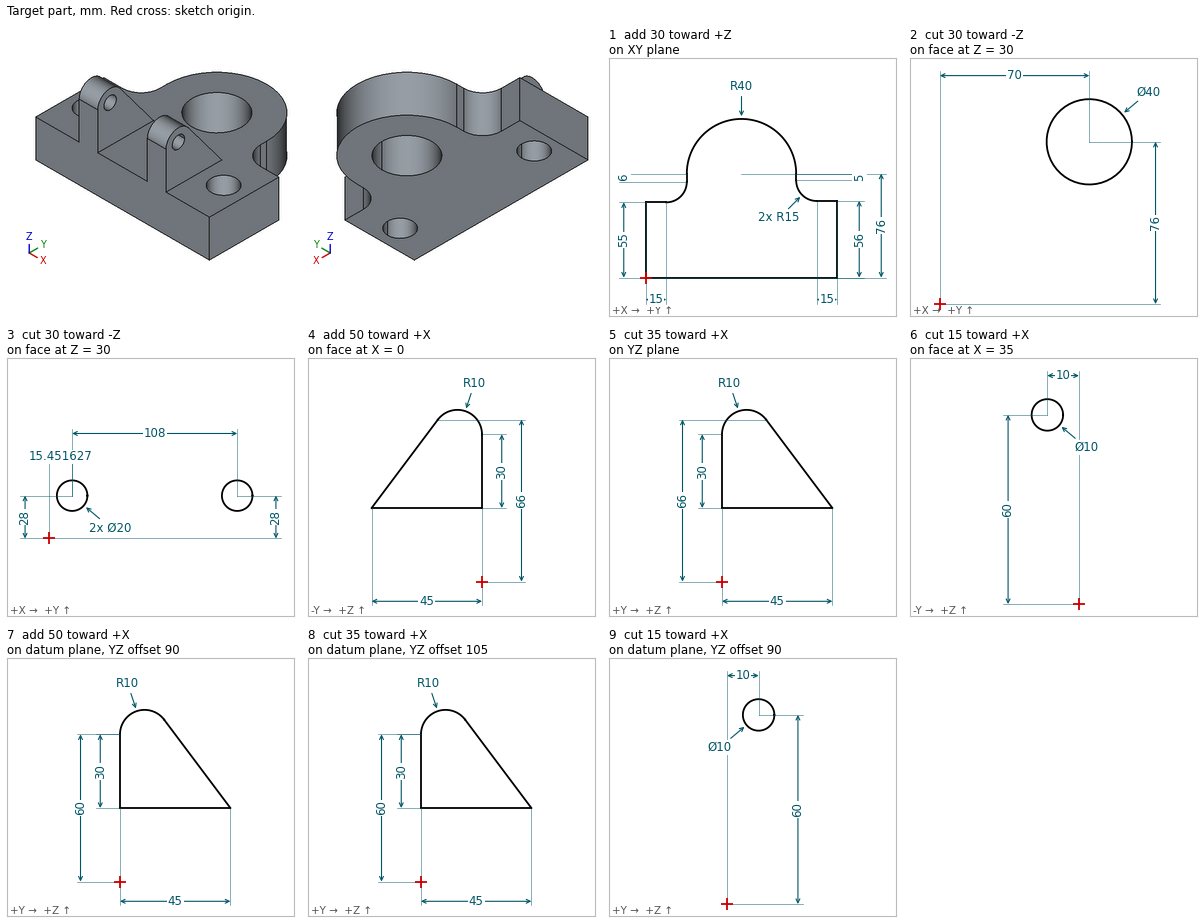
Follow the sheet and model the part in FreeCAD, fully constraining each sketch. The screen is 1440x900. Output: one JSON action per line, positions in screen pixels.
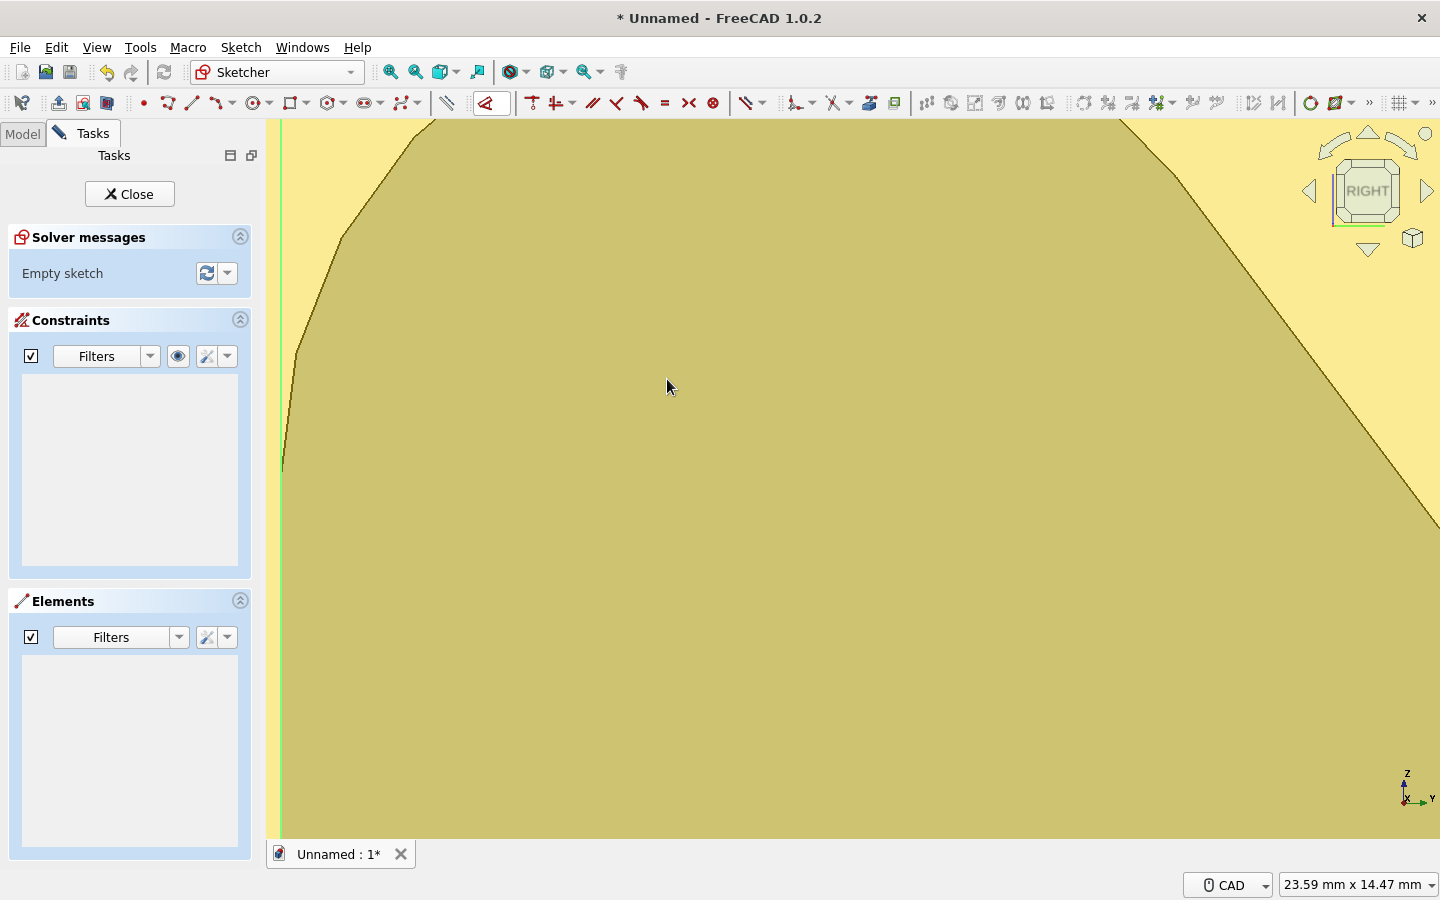
{"action": "key", "text": "g c"}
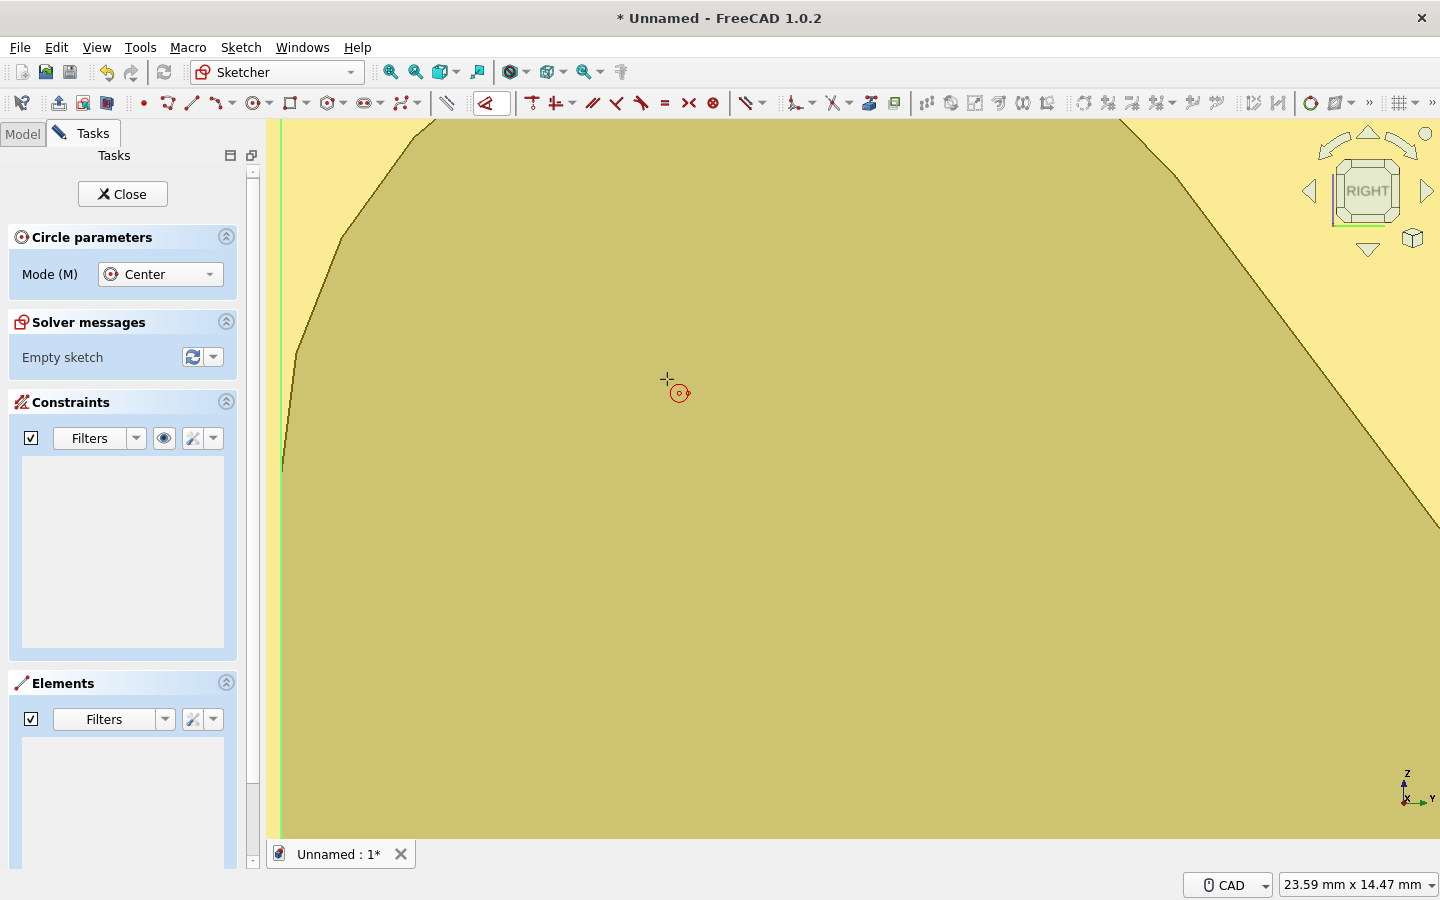
{"action": "left_click", "coordinate": [779, 476]}
{"action": "mouse_move", "coordinate": [954, 300]}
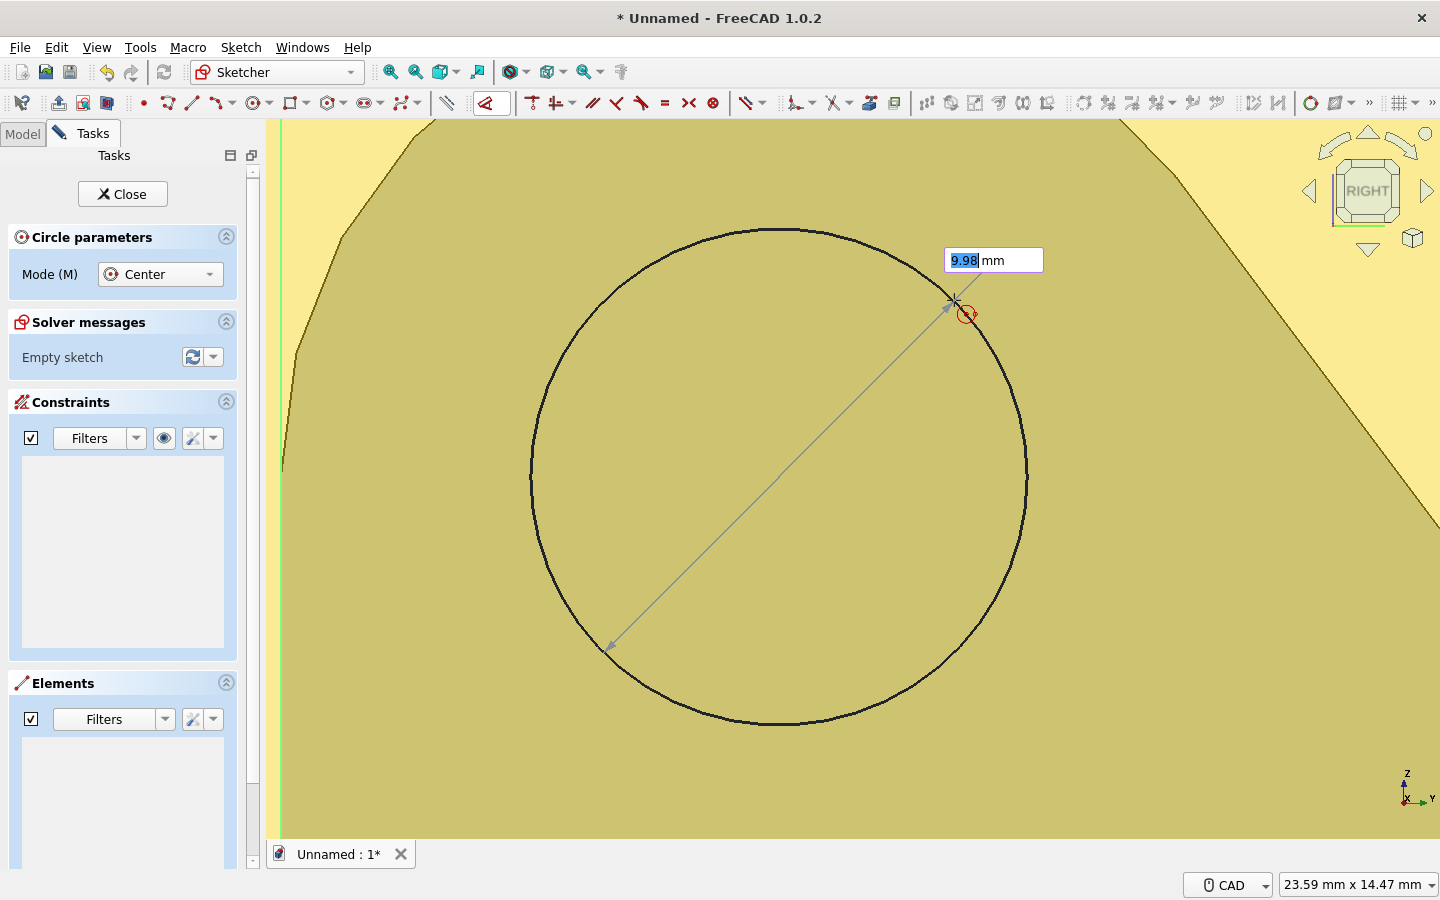
{"action": "type", "text": "10"}
{"action": "key", "text": "Return"}
{"action": "key", "text": "Escape"}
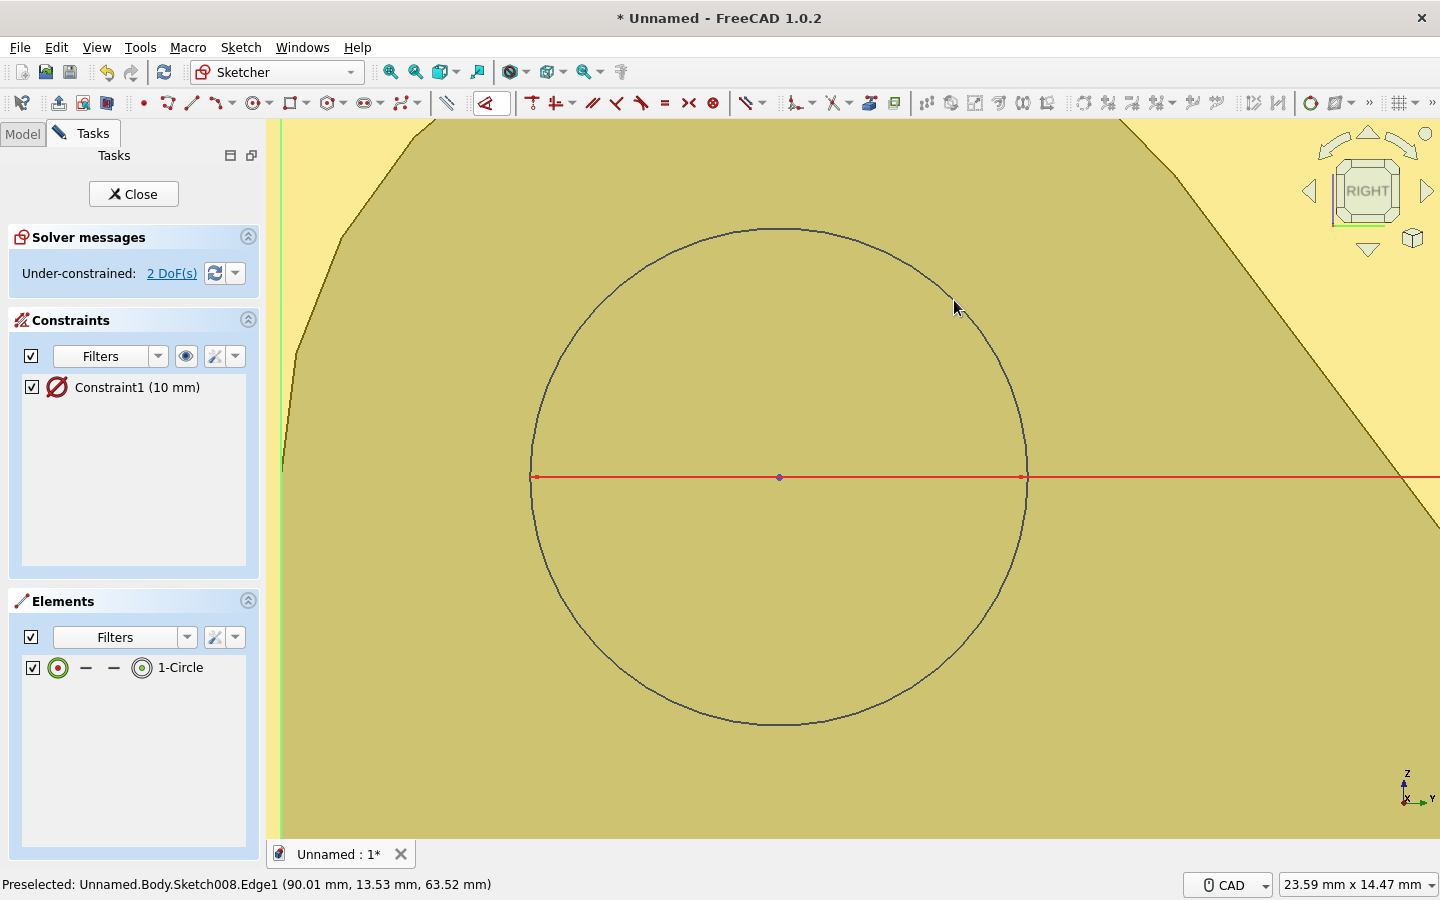
{"action": "left_click", "coordinate": [779, 477]}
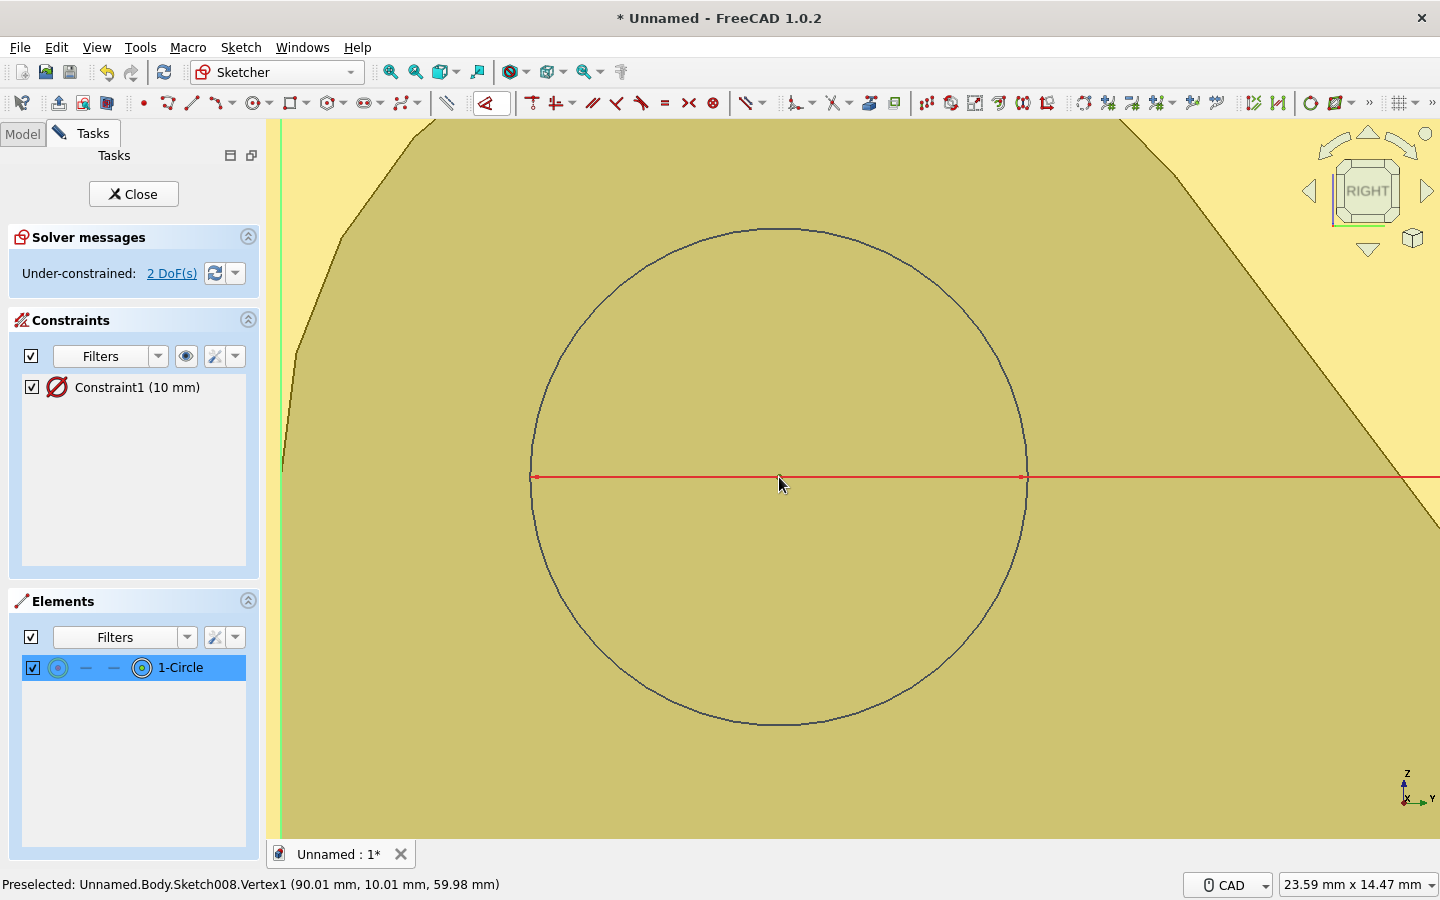
{"action": "key", "text": "l"}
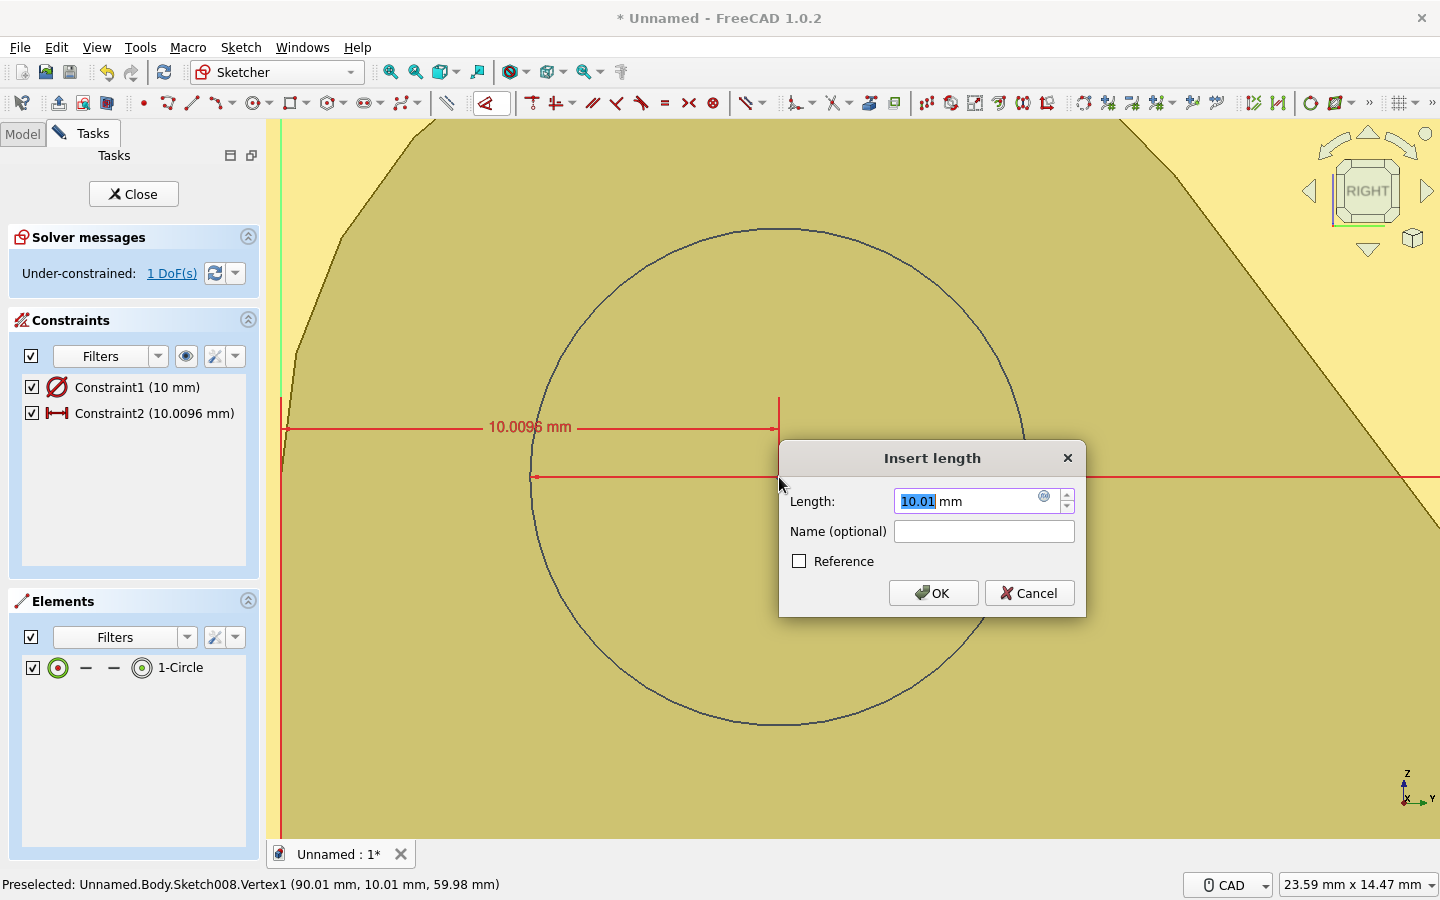
{"action": "type", "text": "10"}
{"action": "key", "text": "Return"}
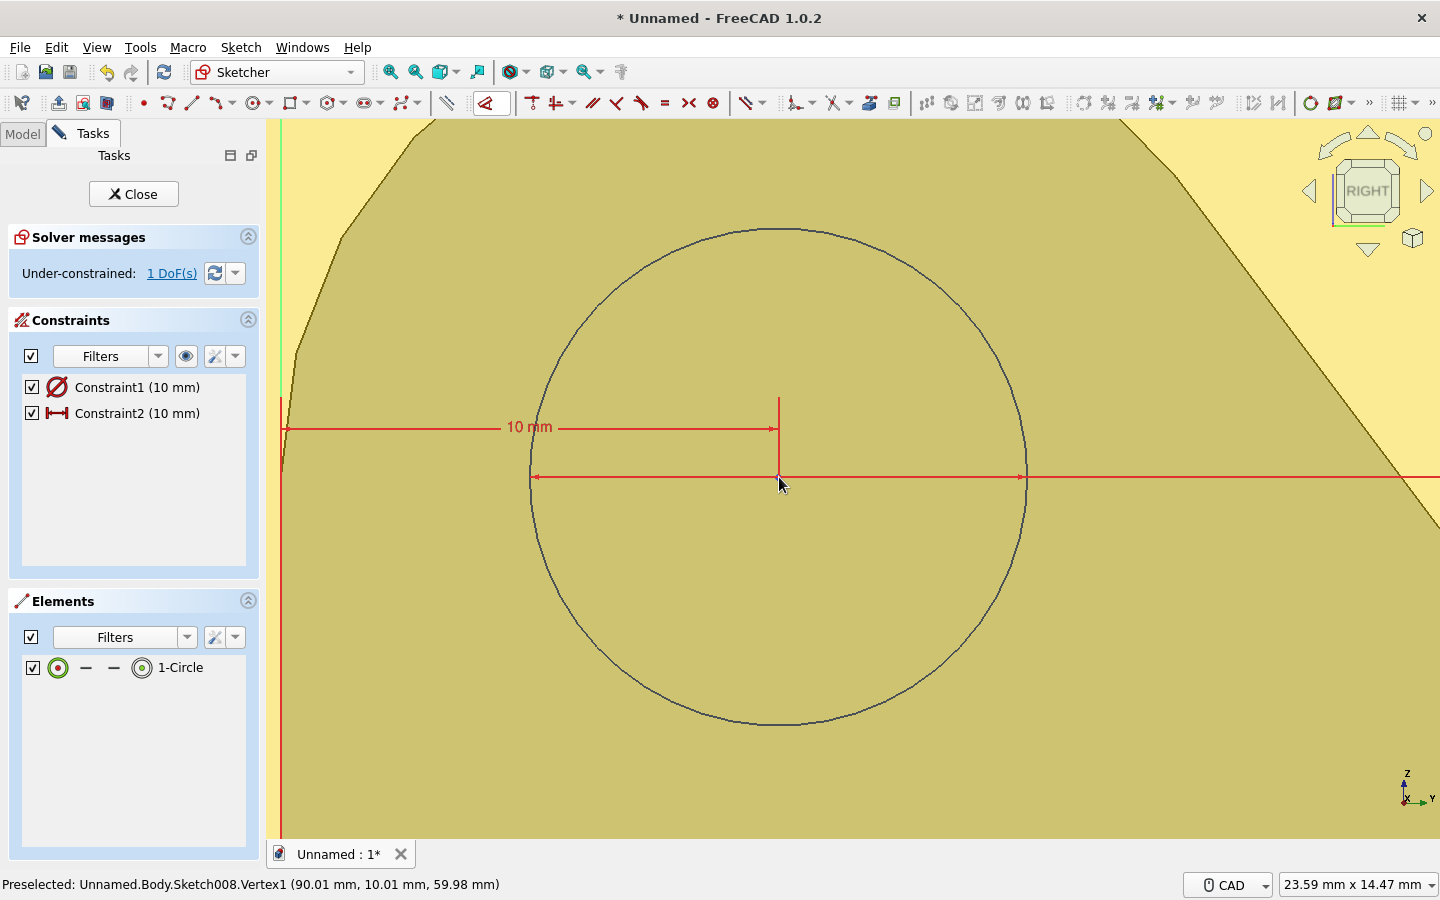
{"action": "left_click", "coordinate": [779, 477]}